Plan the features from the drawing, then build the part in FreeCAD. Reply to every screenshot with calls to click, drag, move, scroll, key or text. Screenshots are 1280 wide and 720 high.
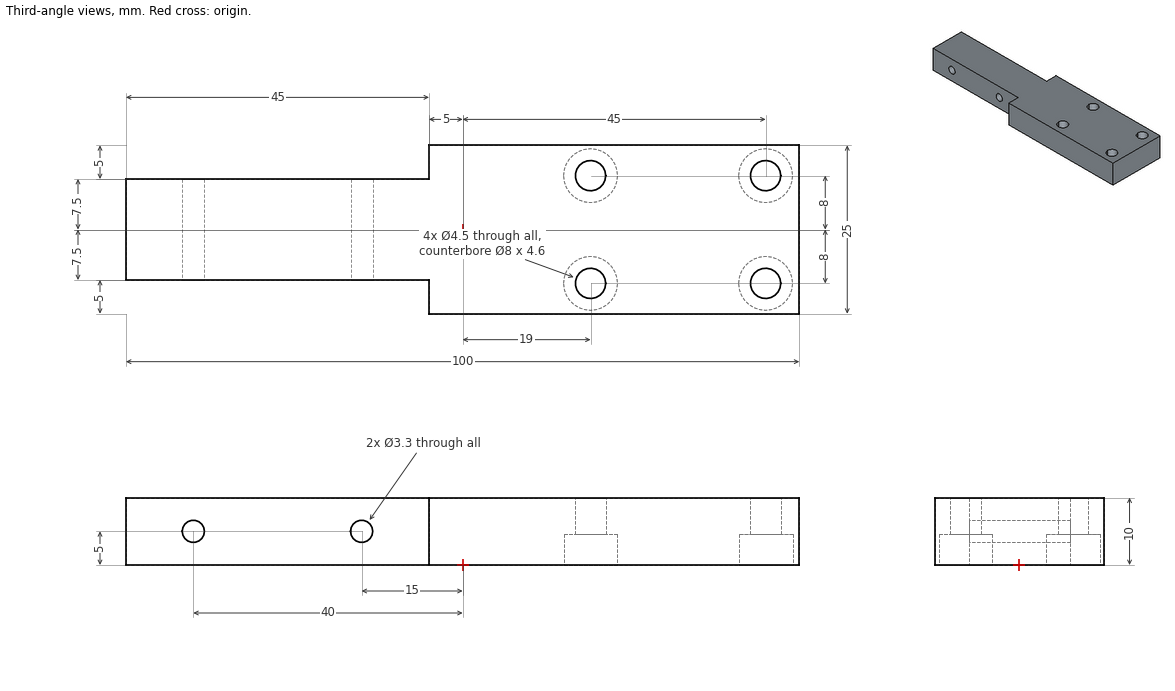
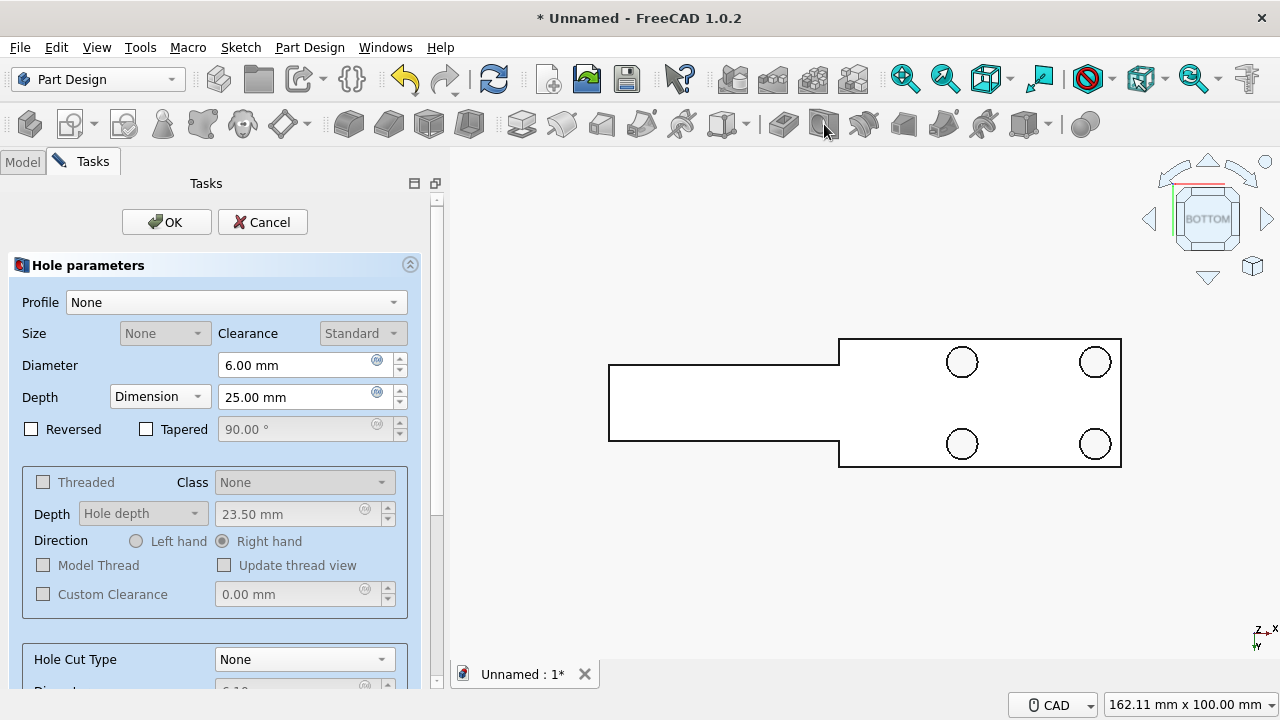
triple_click(305, 365)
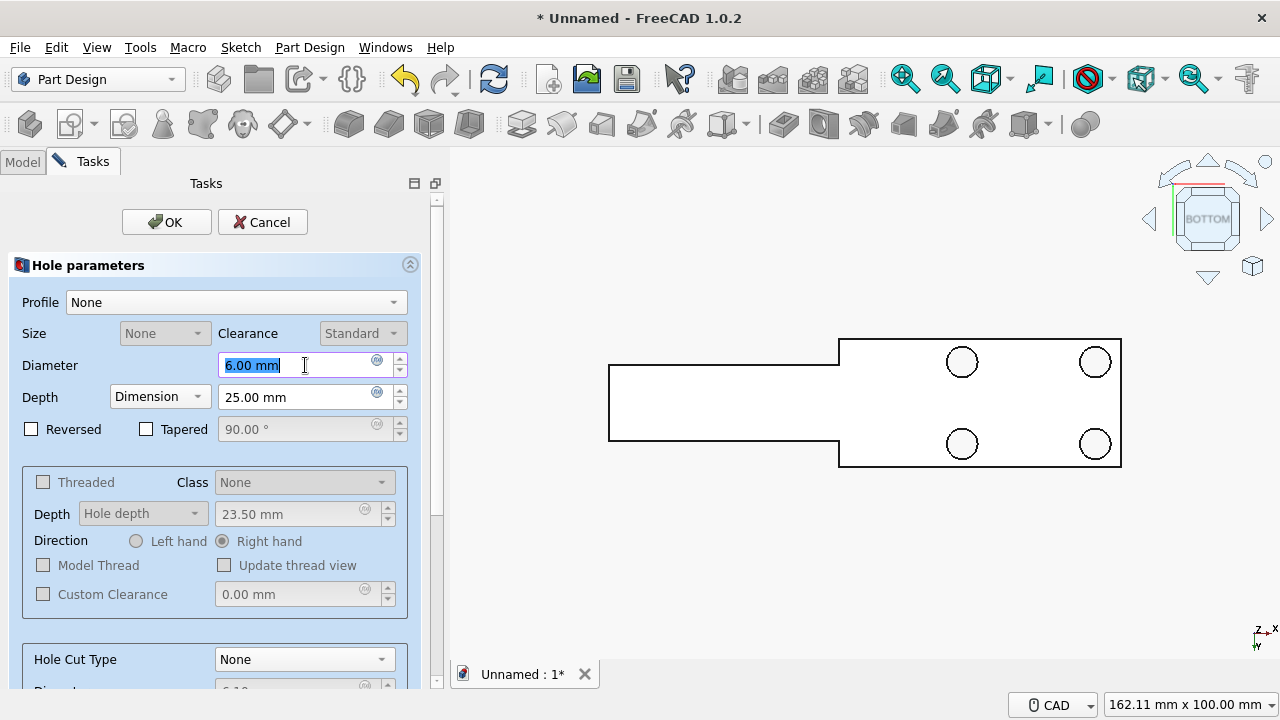
text(4.5)
key(Tab)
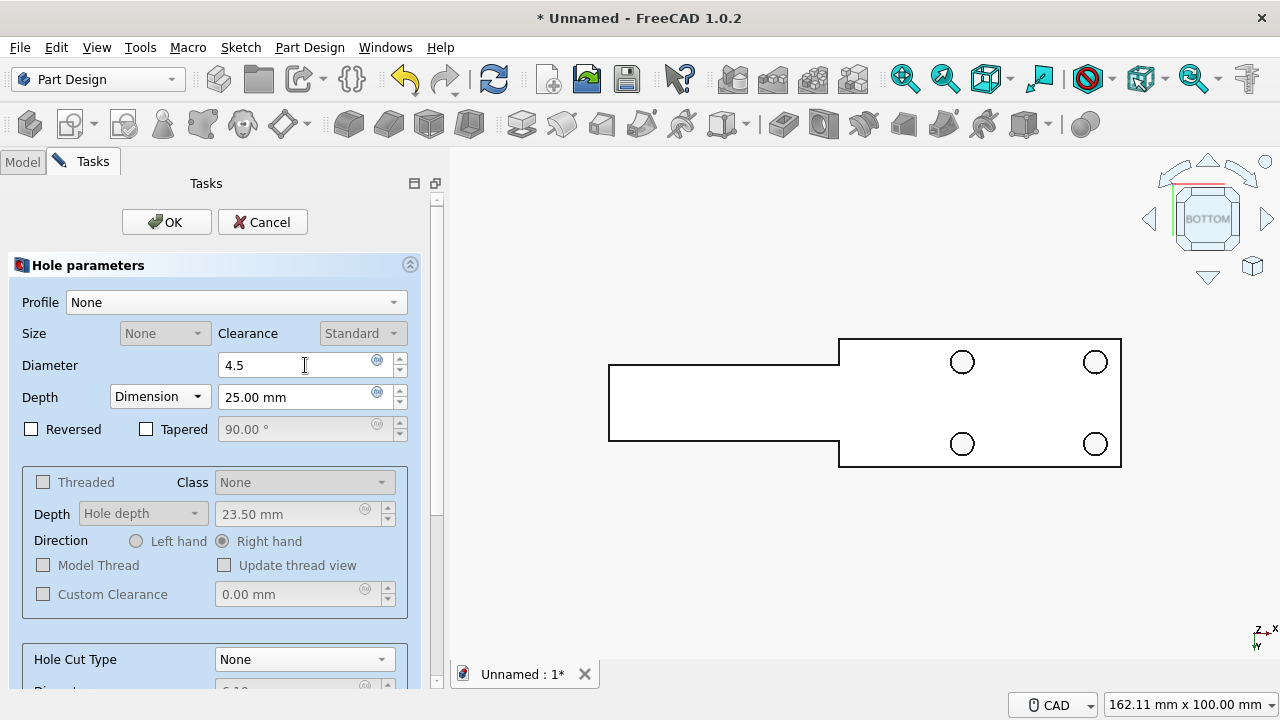
click(161, 396)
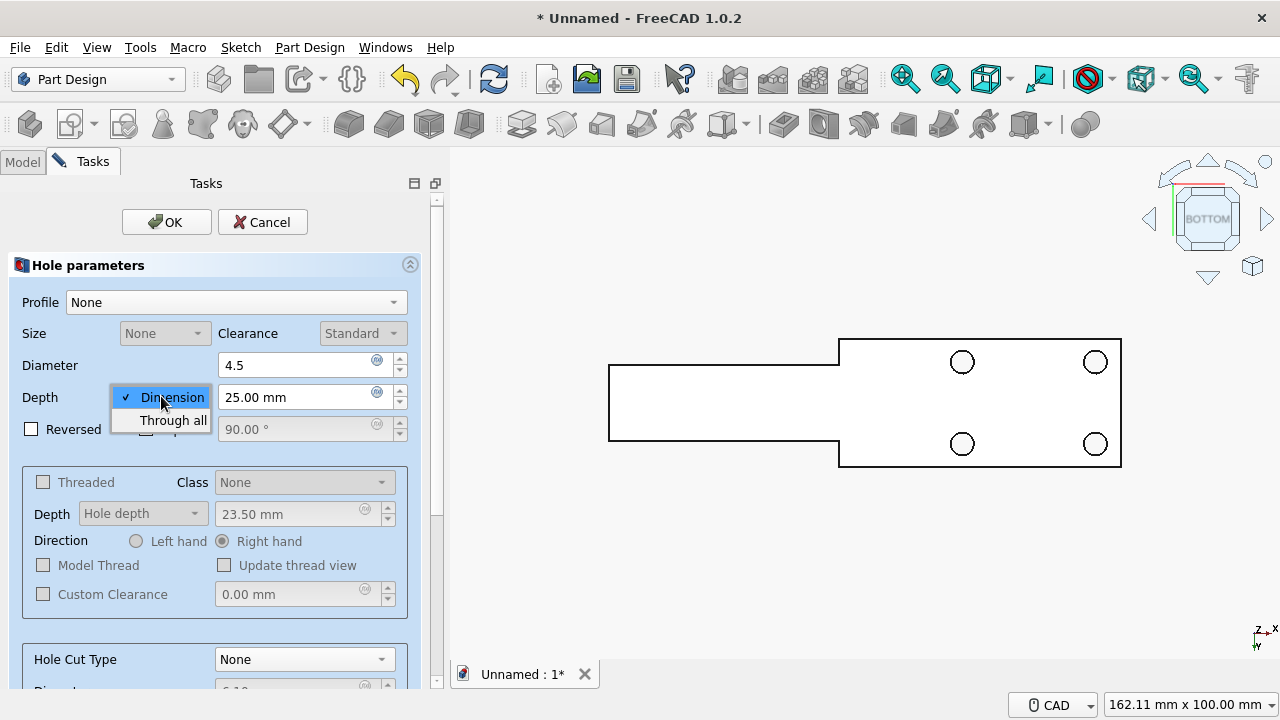
click(160, 420)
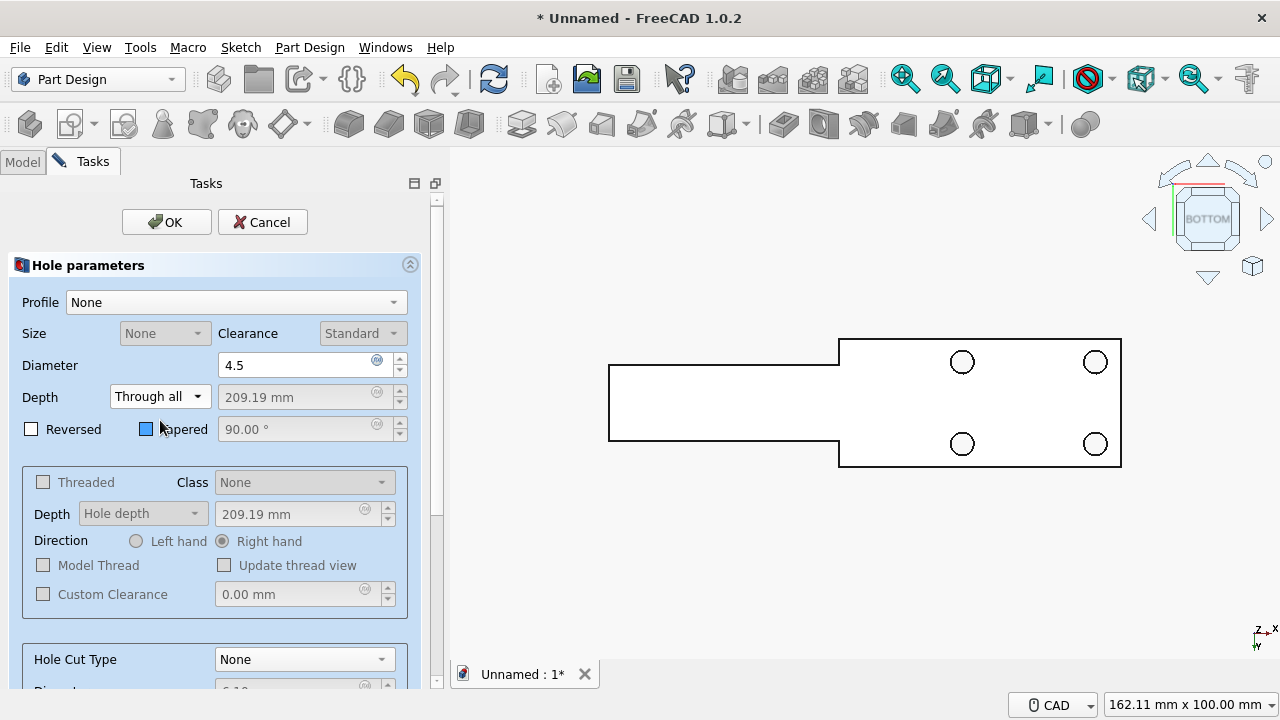
click(306, 660)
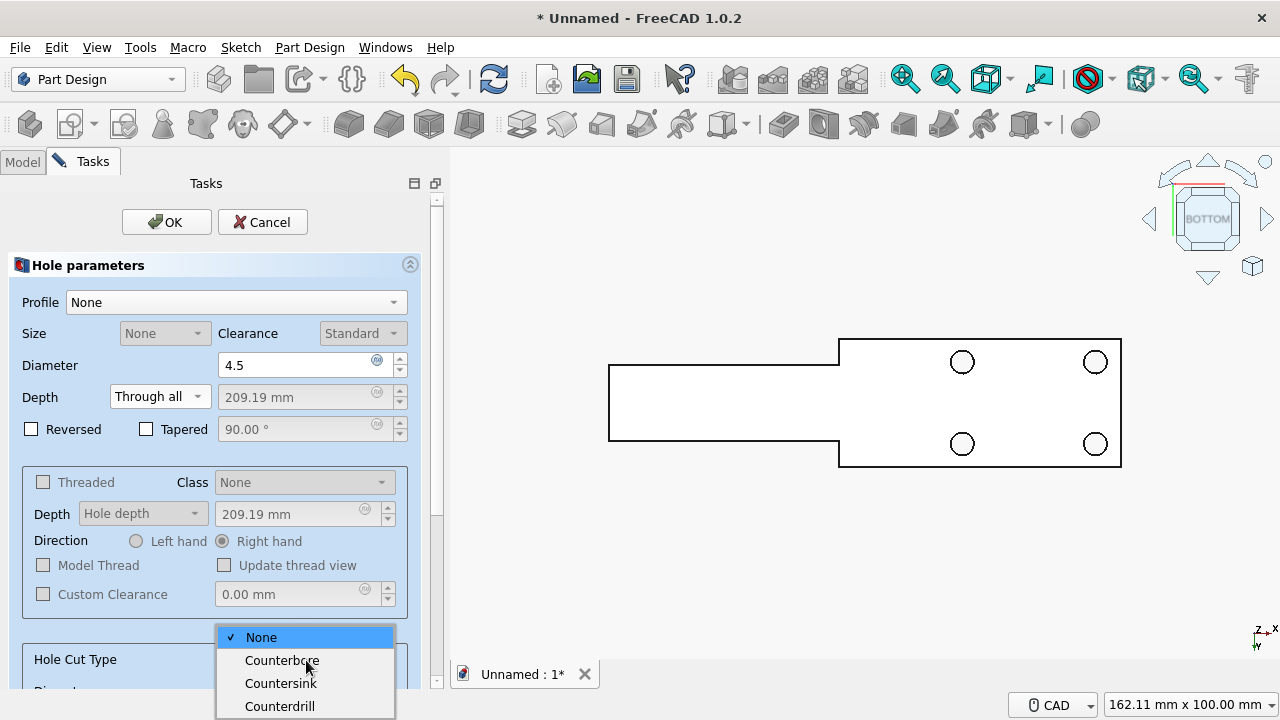
click(304, 660)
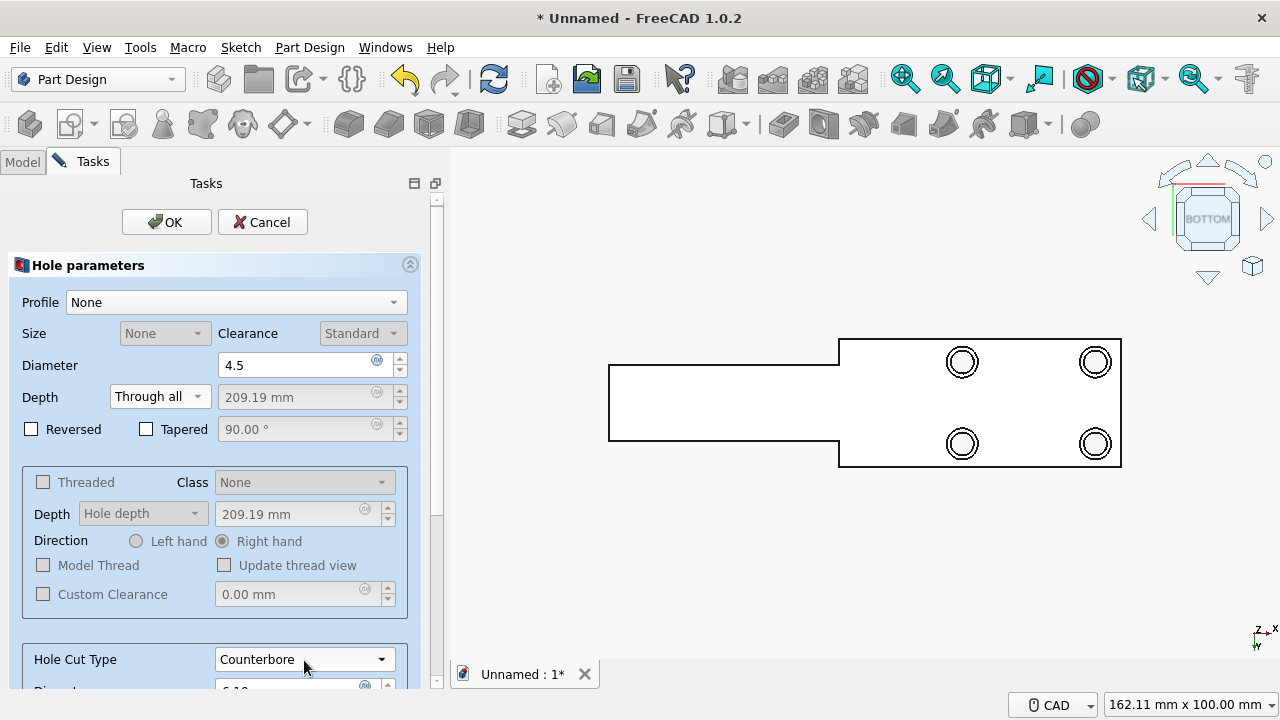
scroll(437, 440, down, 2)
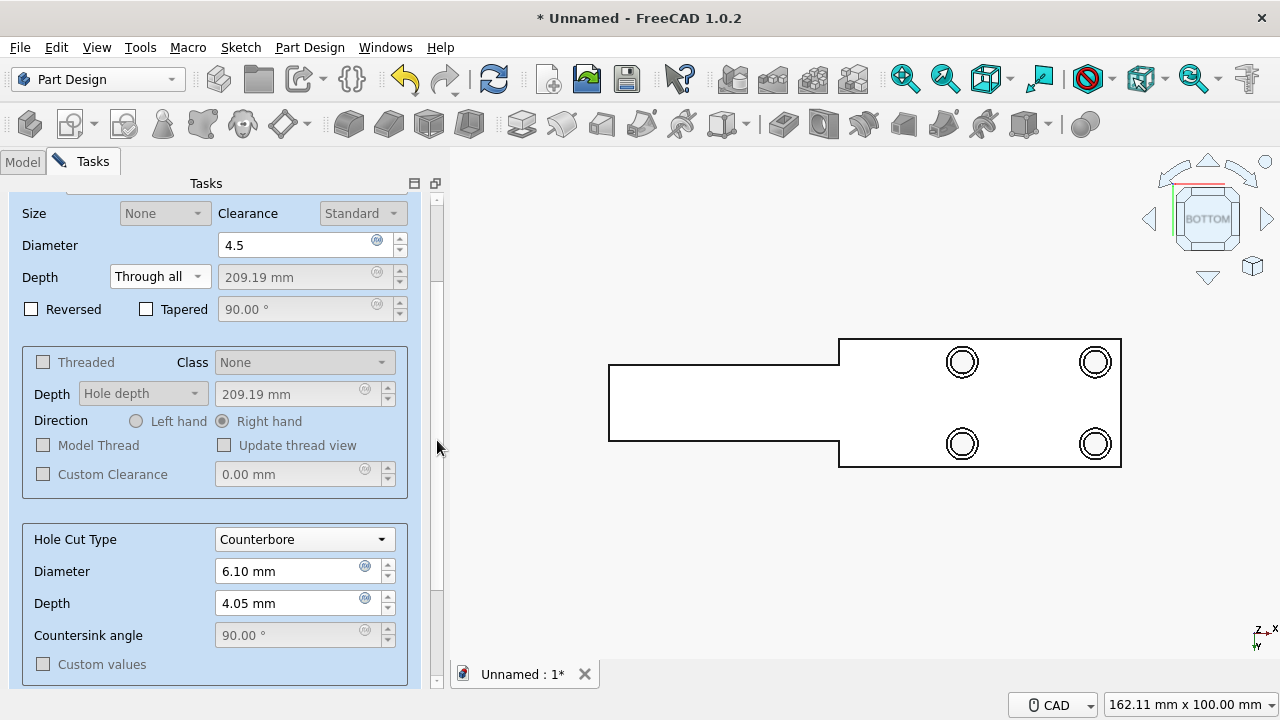
triple_click(298, 571)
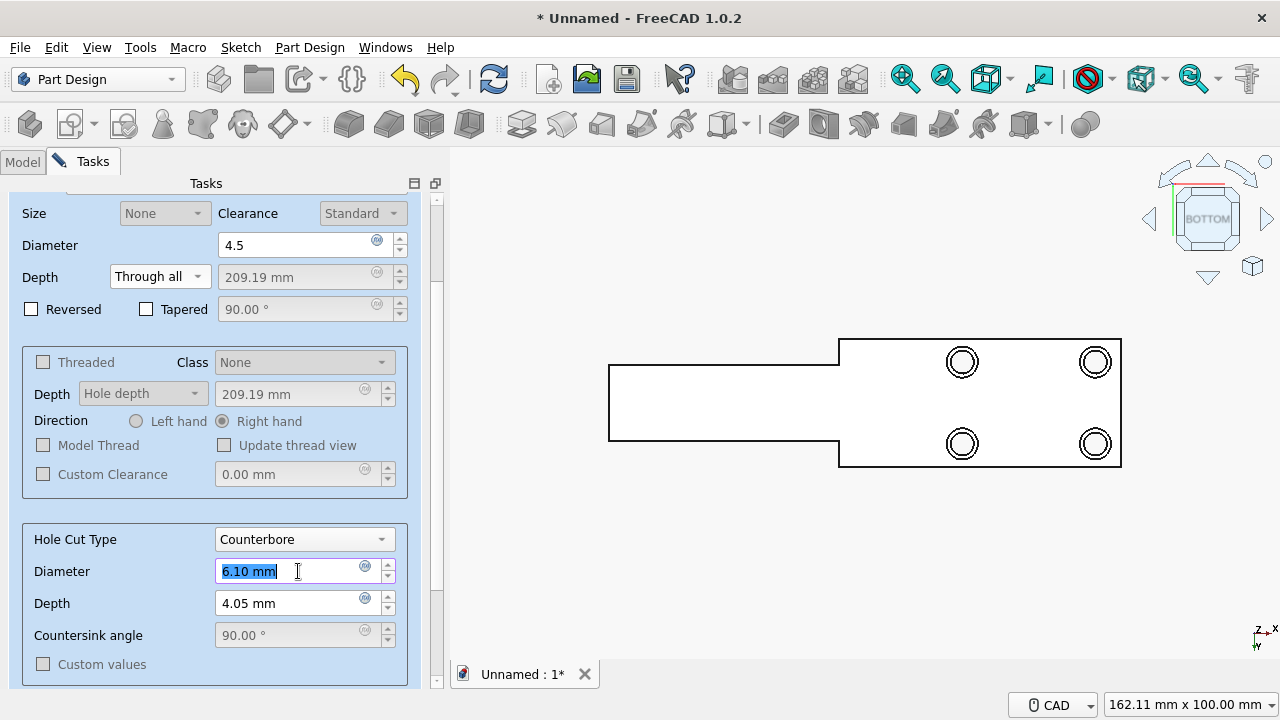
text(8)
key(Tab)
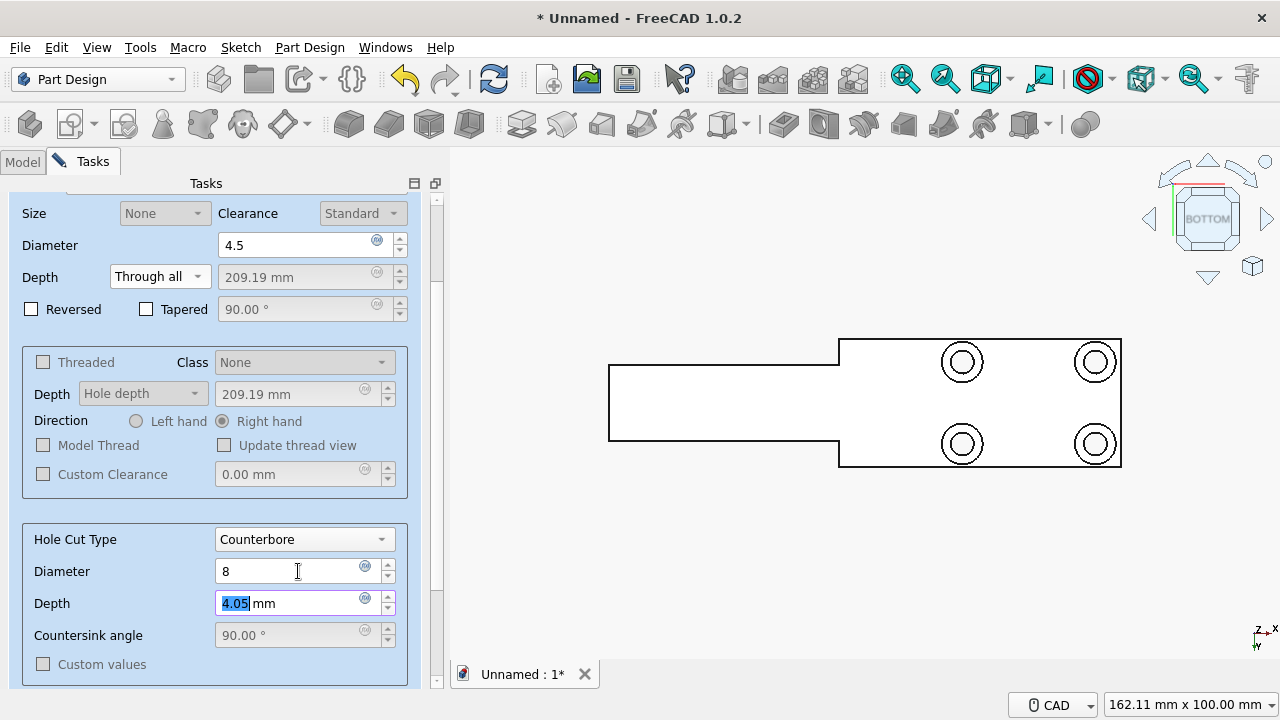
text(4.6)
key(Tab)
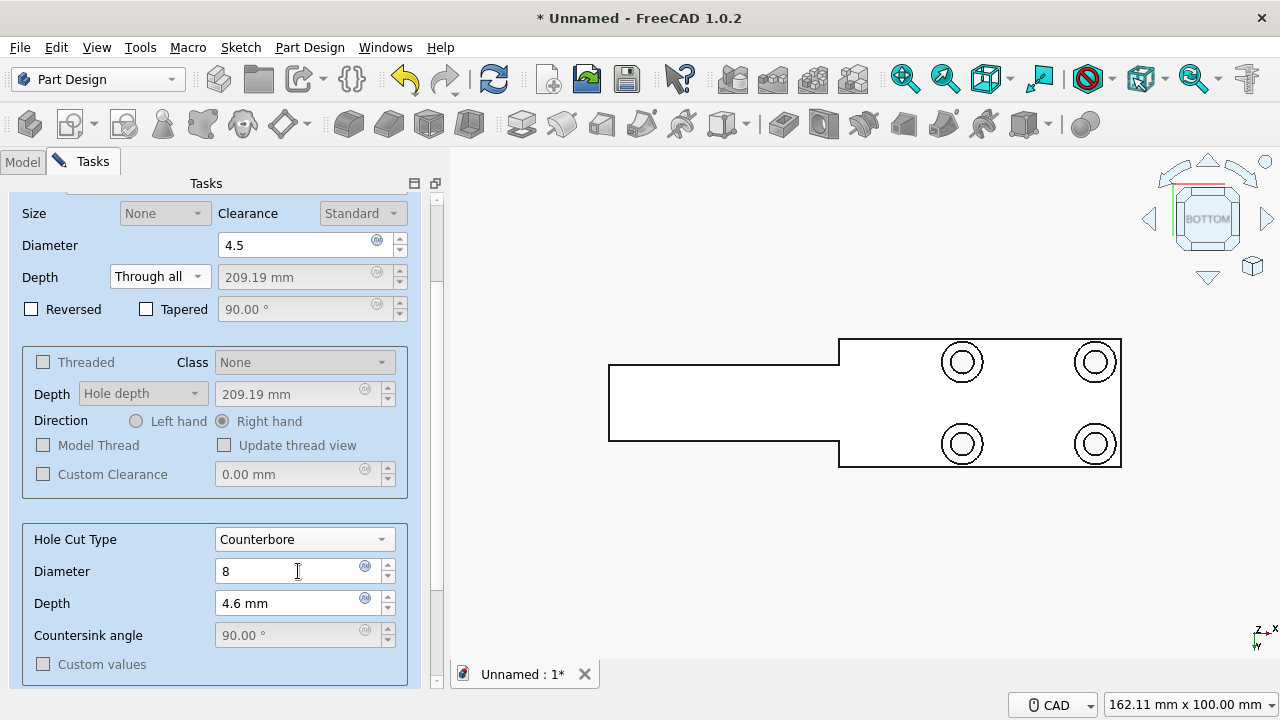
scroll(437, 440, up, 3)